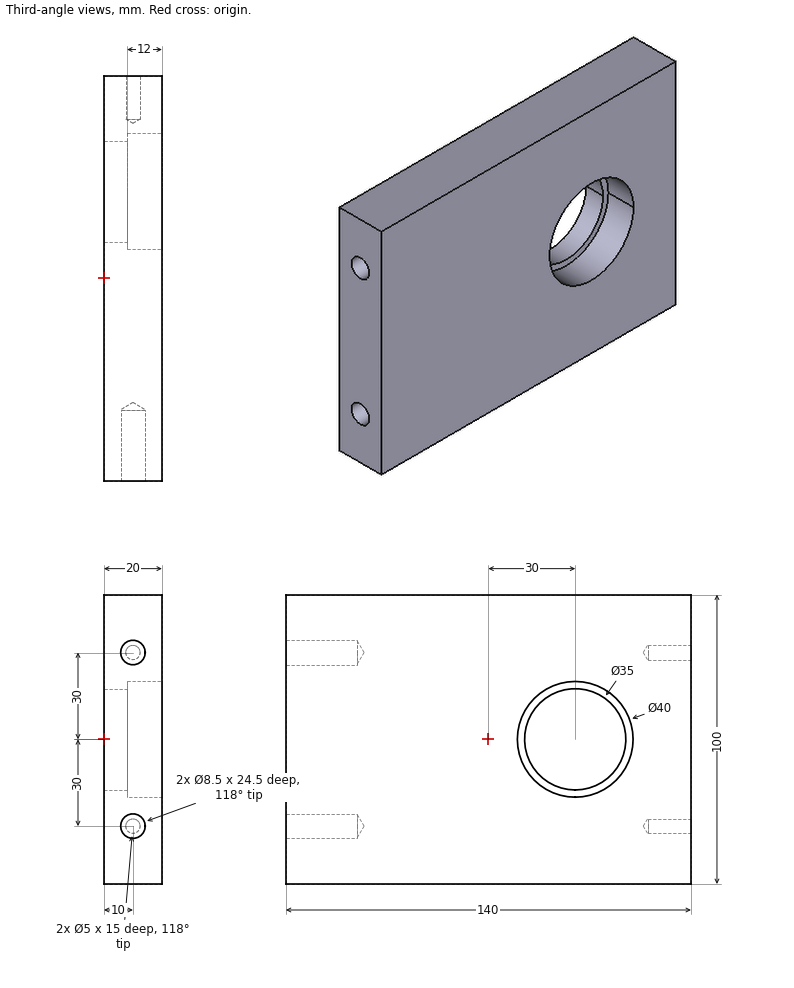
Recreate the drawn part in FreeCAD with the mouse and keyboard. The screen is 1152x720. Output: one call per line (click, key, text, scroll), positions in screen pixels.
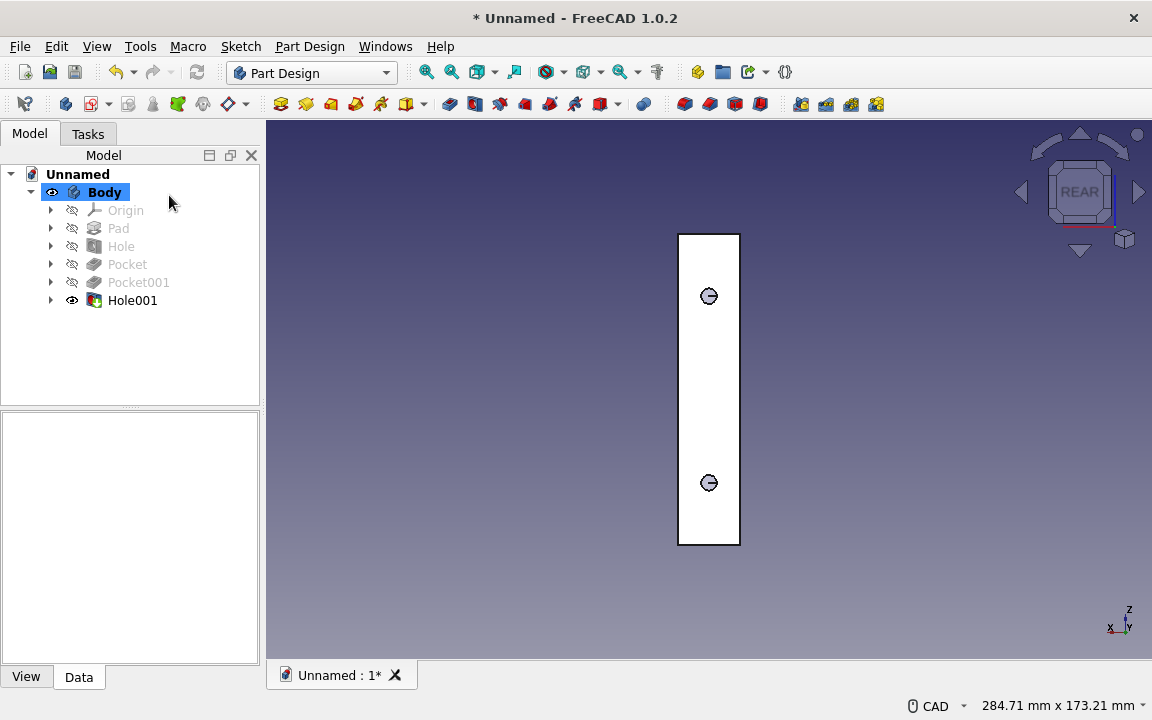
key(0)